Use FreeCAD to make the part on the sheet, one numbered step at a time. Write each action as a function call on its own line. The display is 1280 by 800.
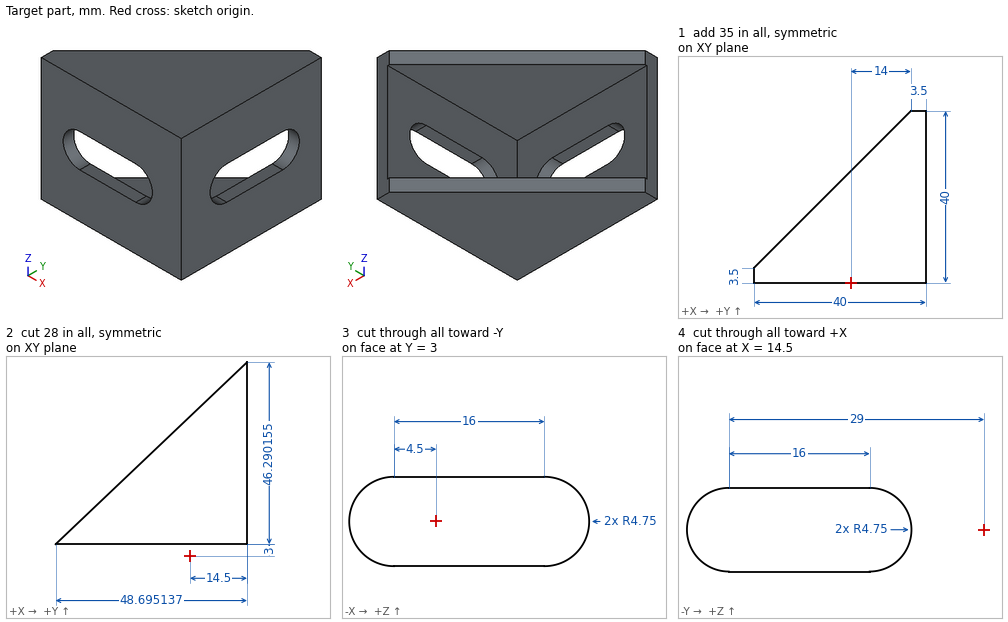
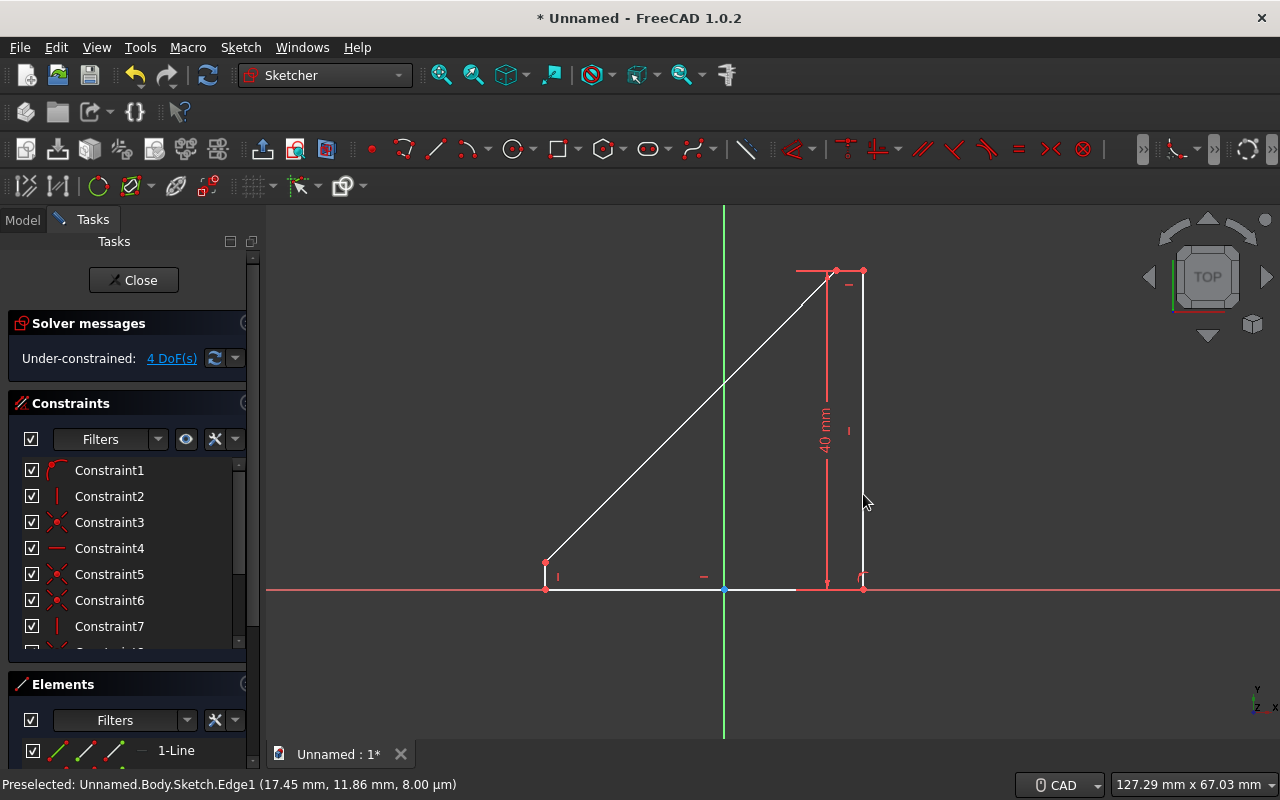
click(640, 590)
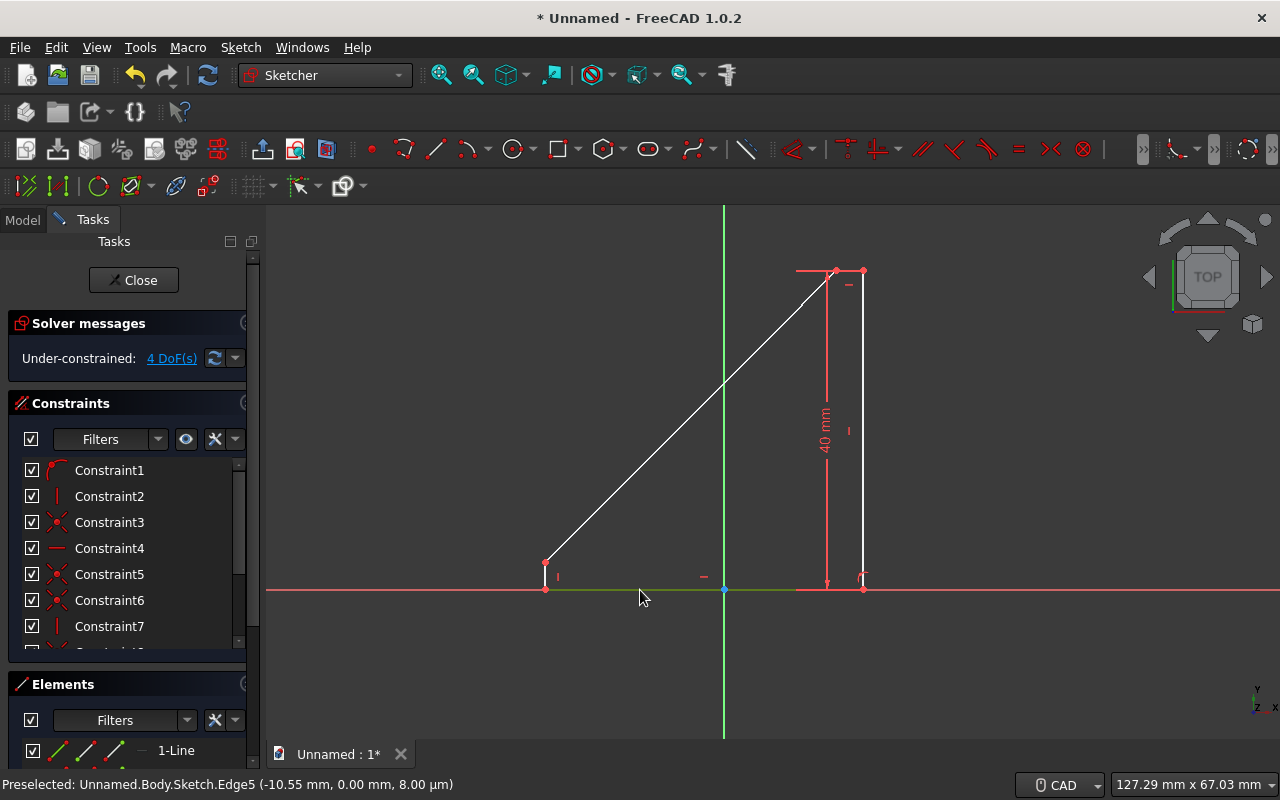
click(814, 150)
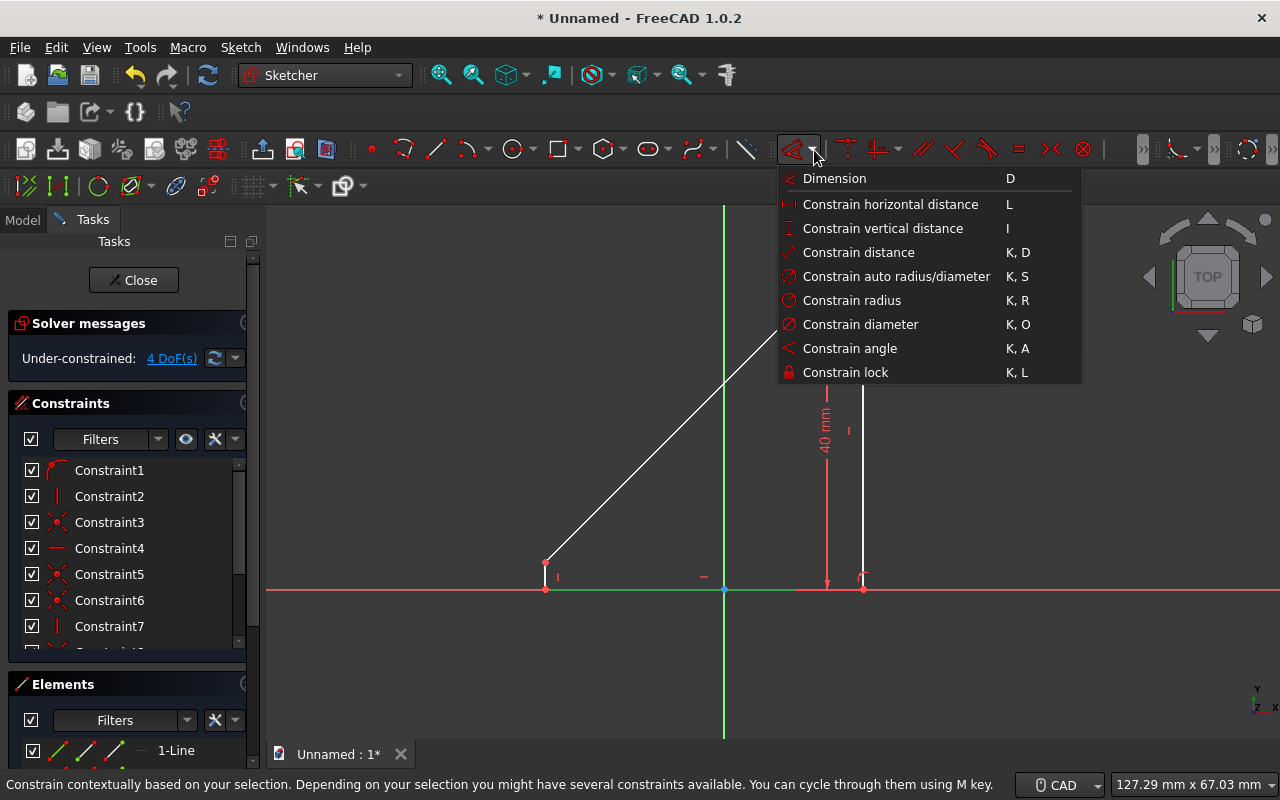
click(930, 204)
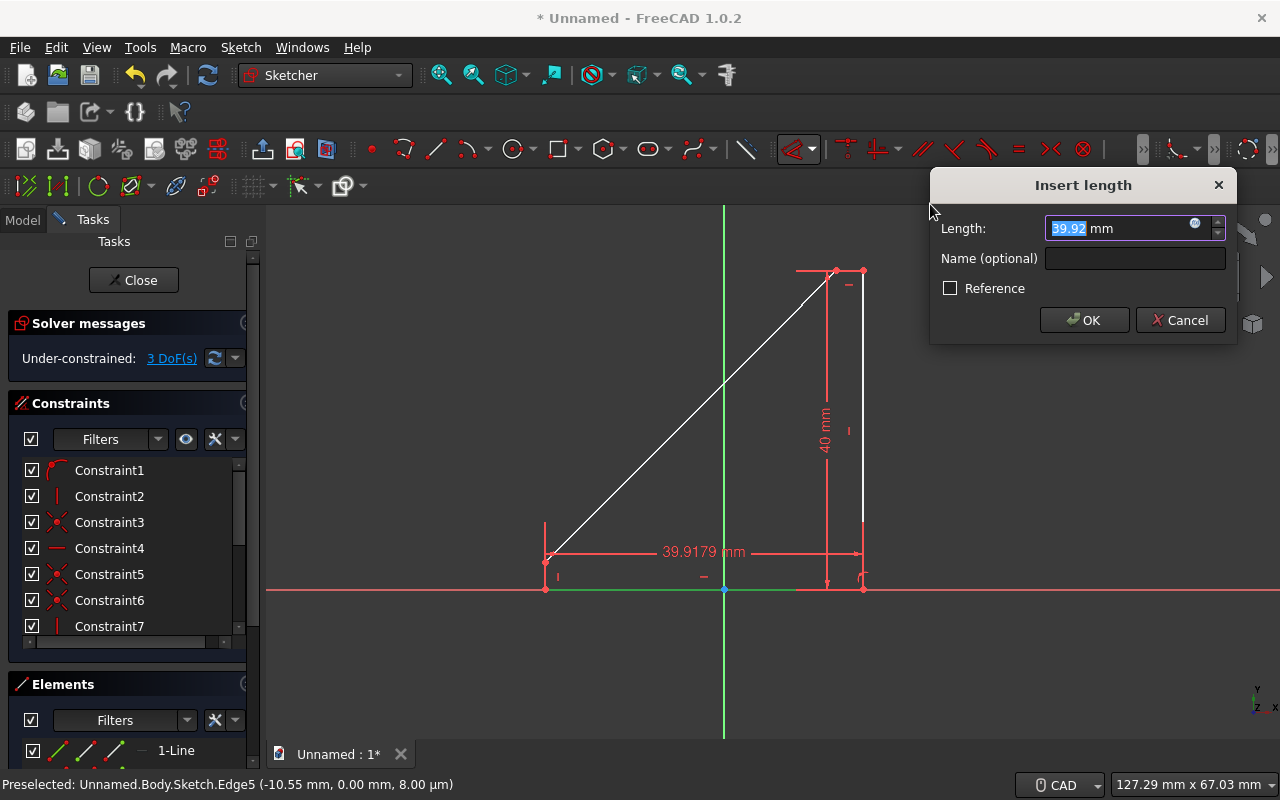
text(40)
key(Return)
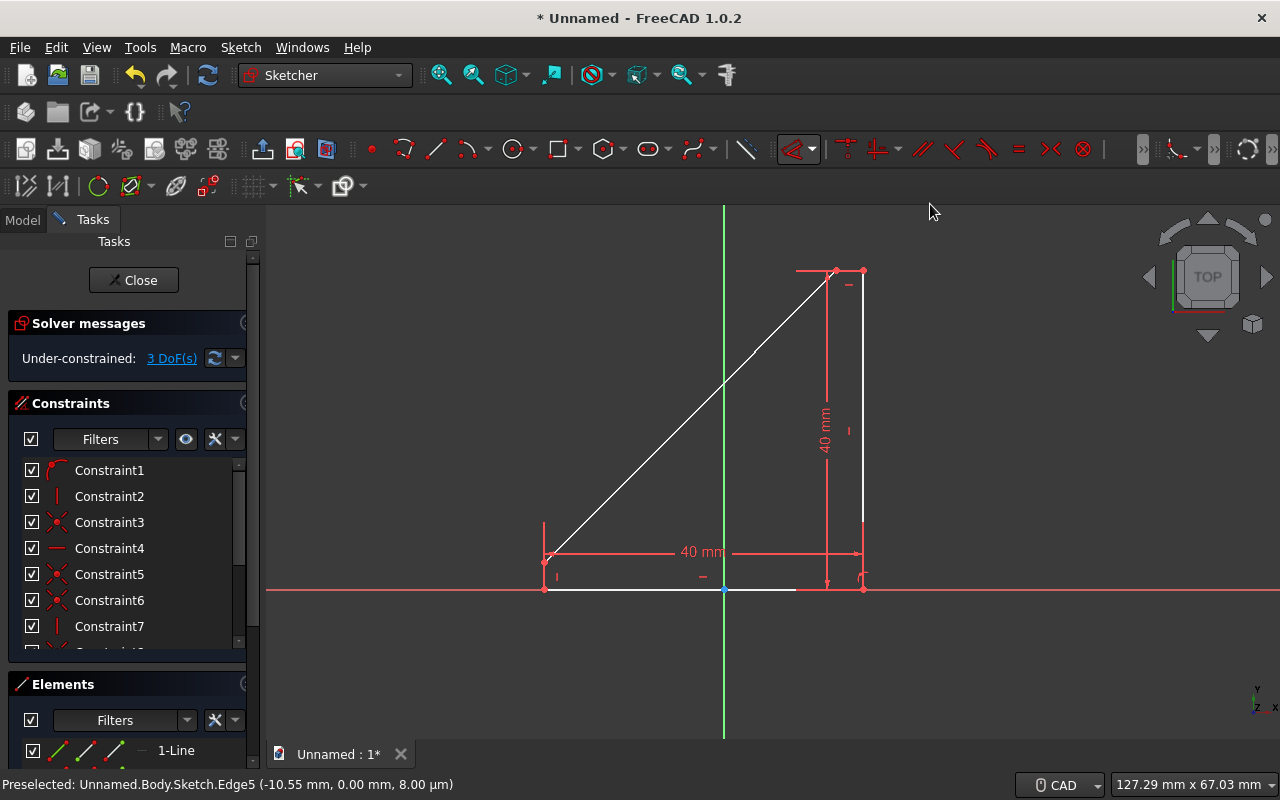
scroll(852, 271, up, 2)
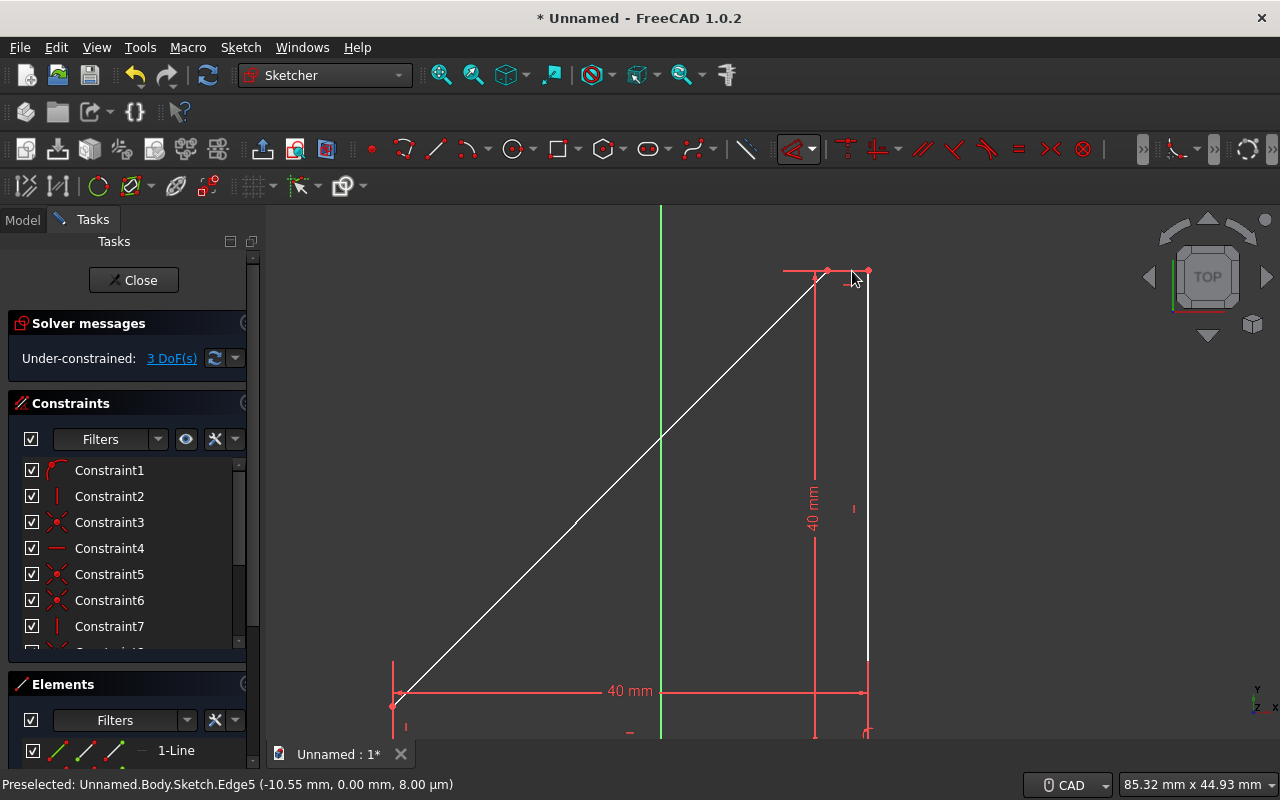
click(852, 271)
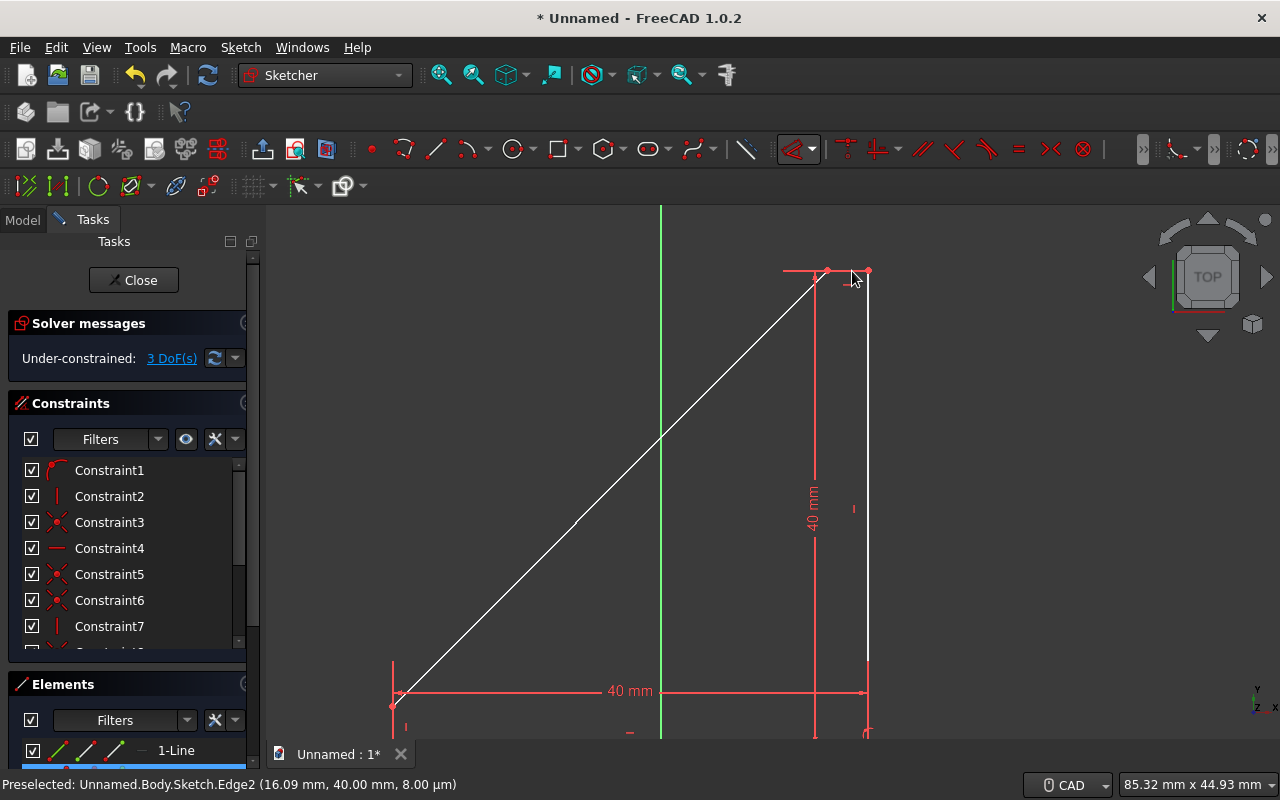
click(814, 150)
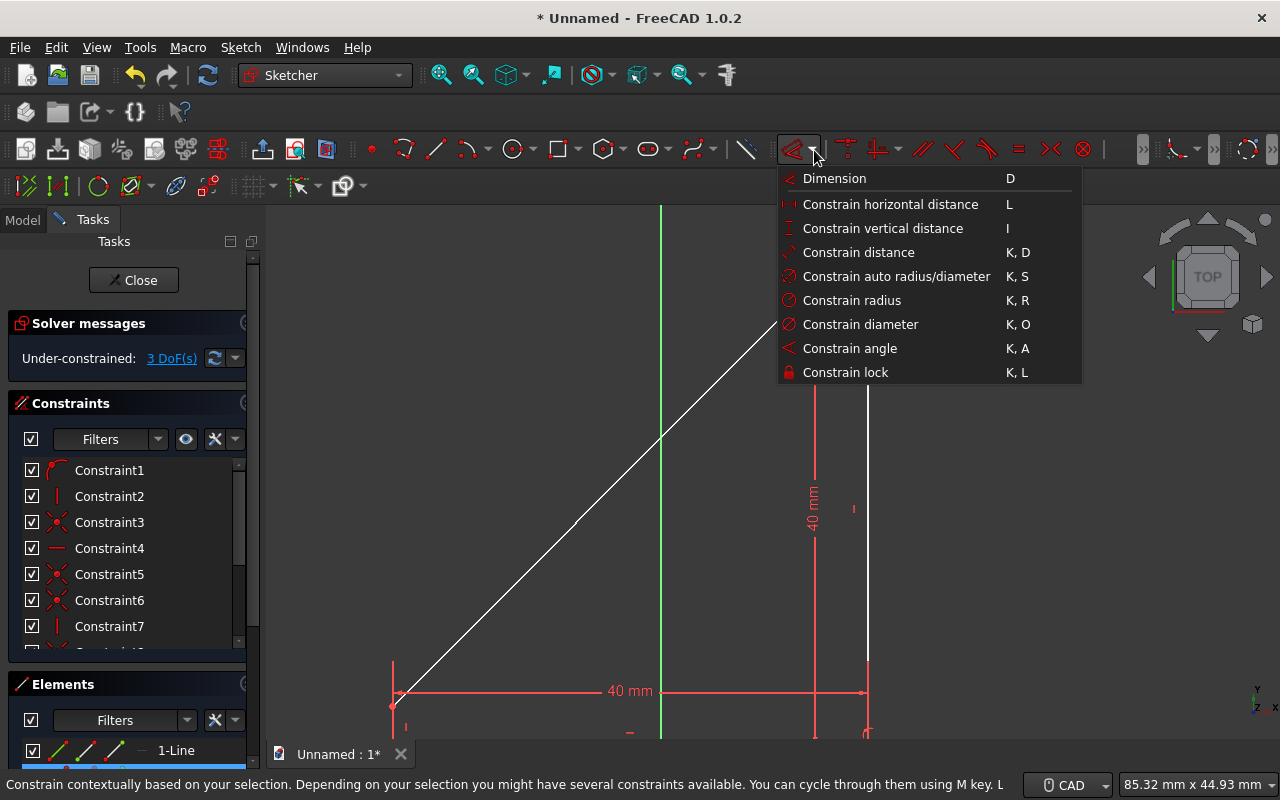
click(930, 204)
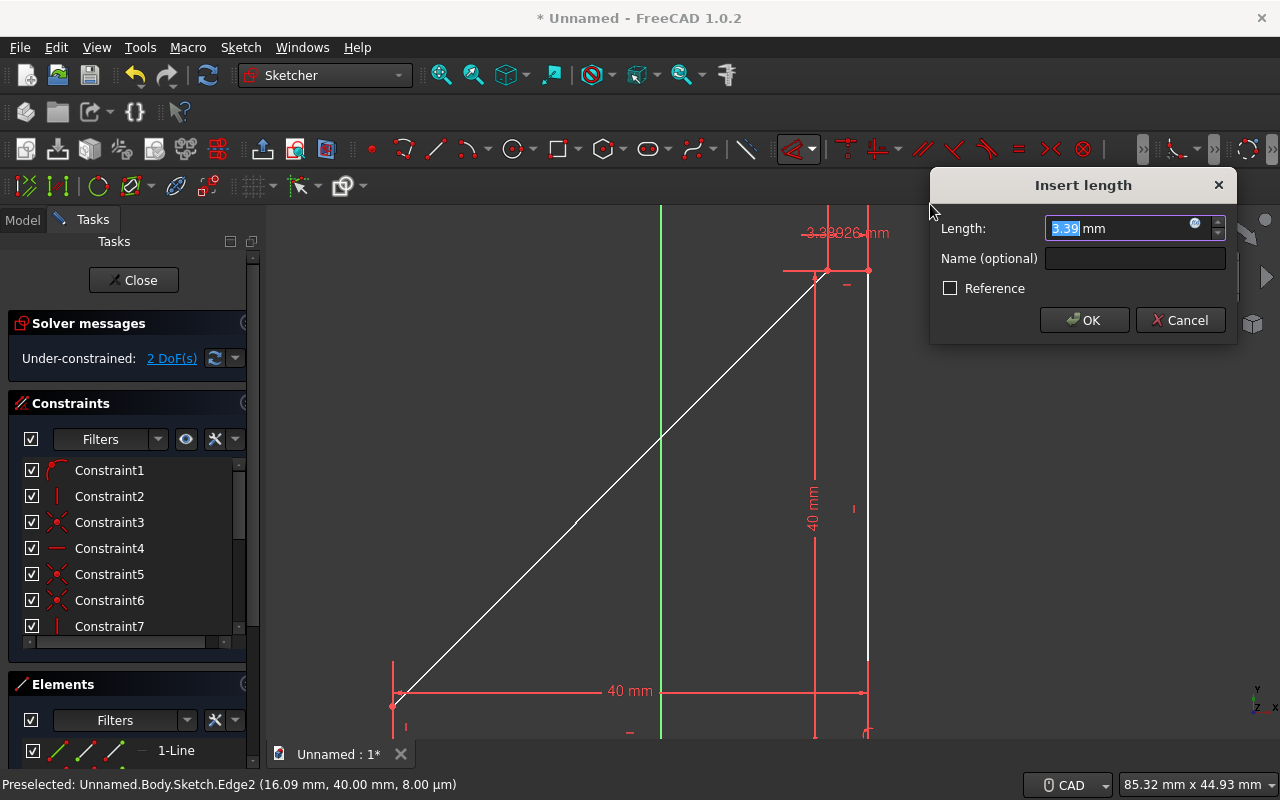
text(3.5)
key(Return)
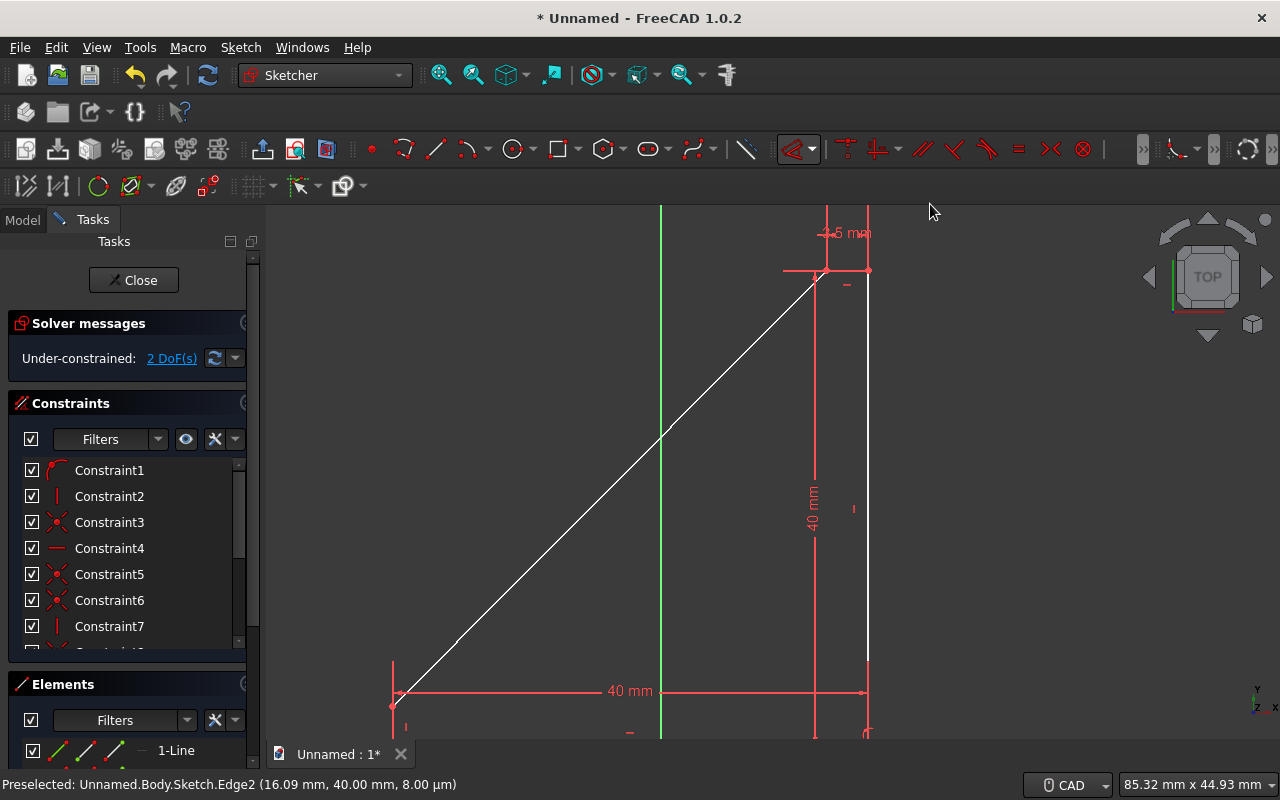
scroll(854, 398, down, 2)